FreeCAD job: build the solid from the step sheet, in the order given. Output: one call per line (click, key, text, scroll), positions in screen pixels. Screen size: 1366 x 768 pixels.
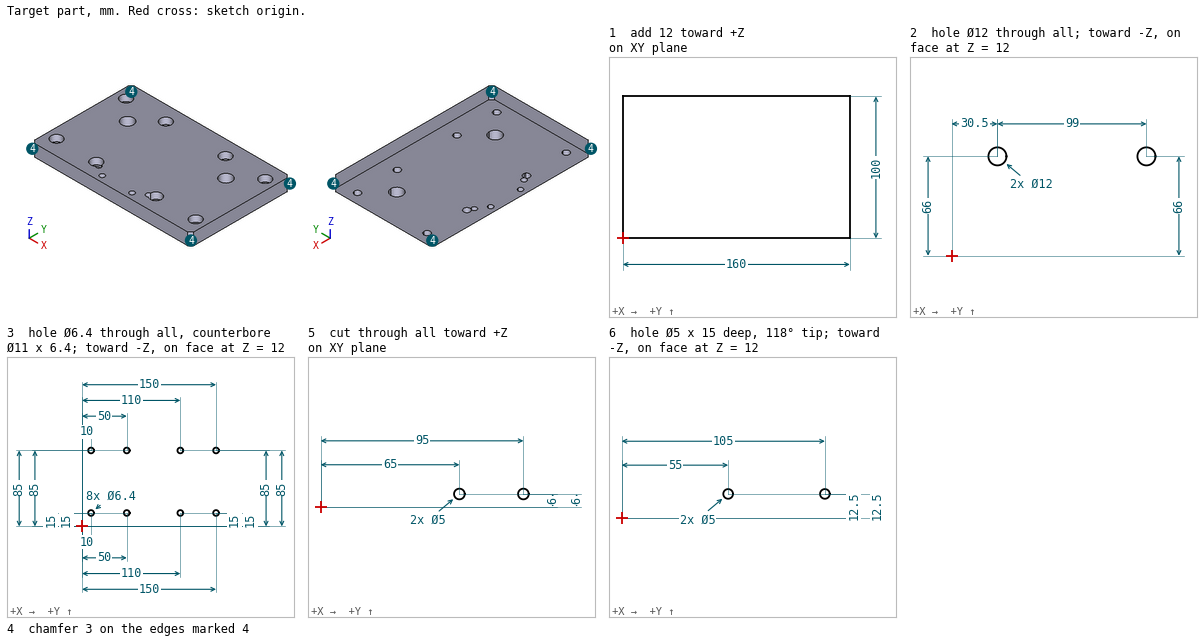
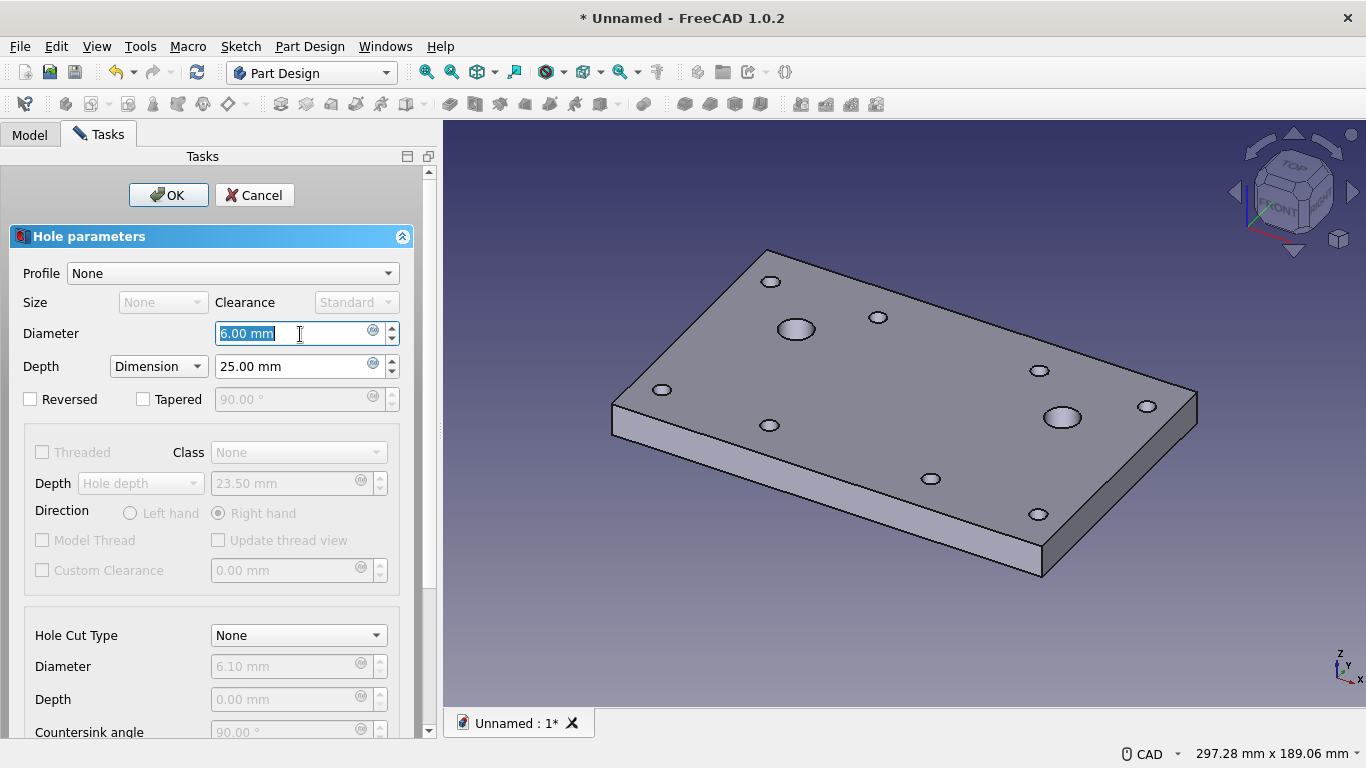
text(6.4)
key(Tab)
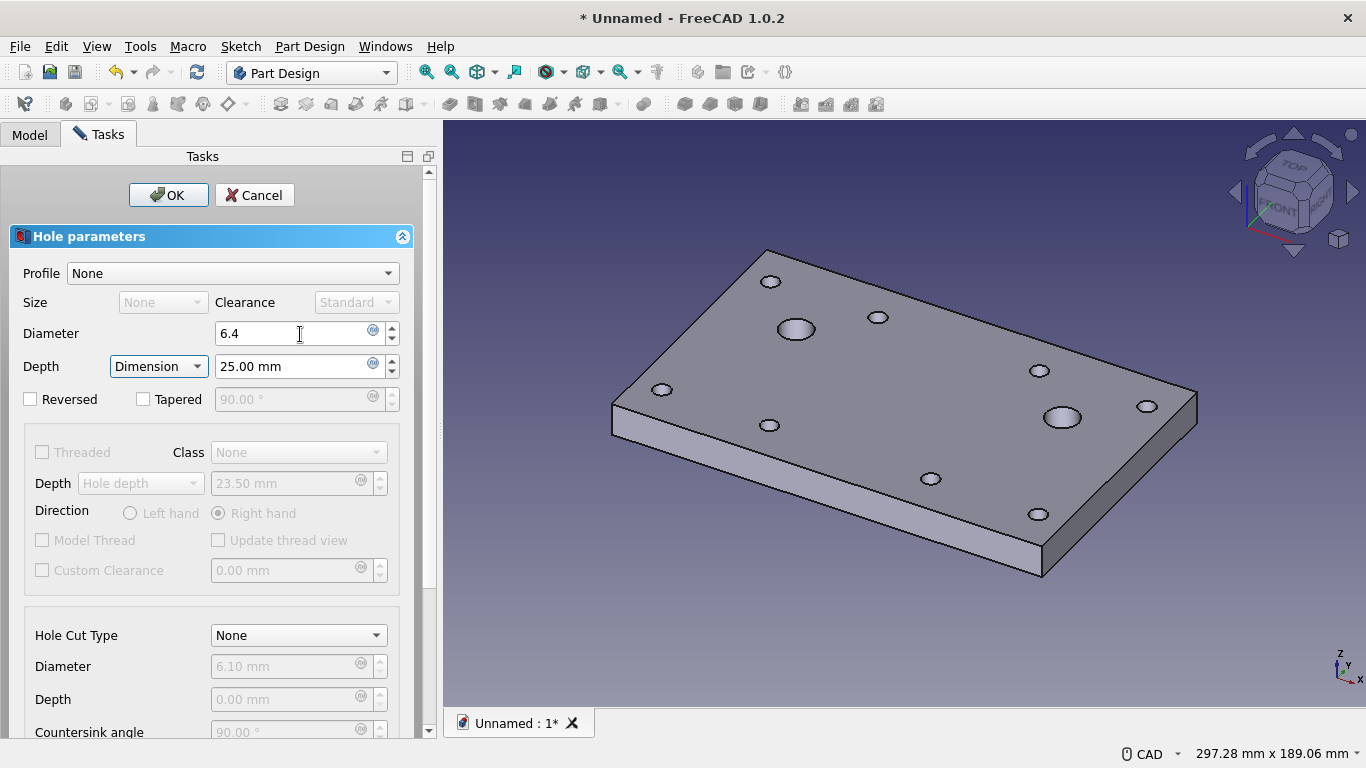
click(160, 366)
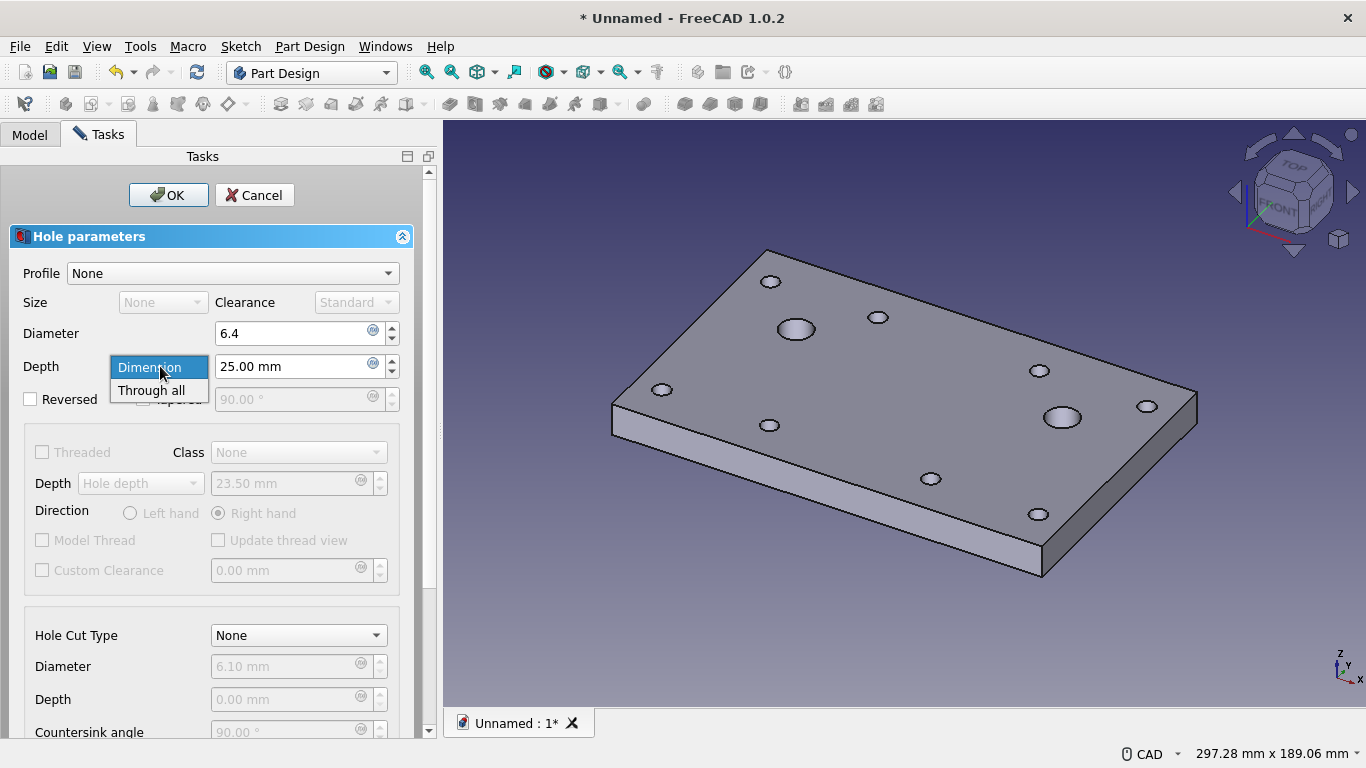
click(158, 390)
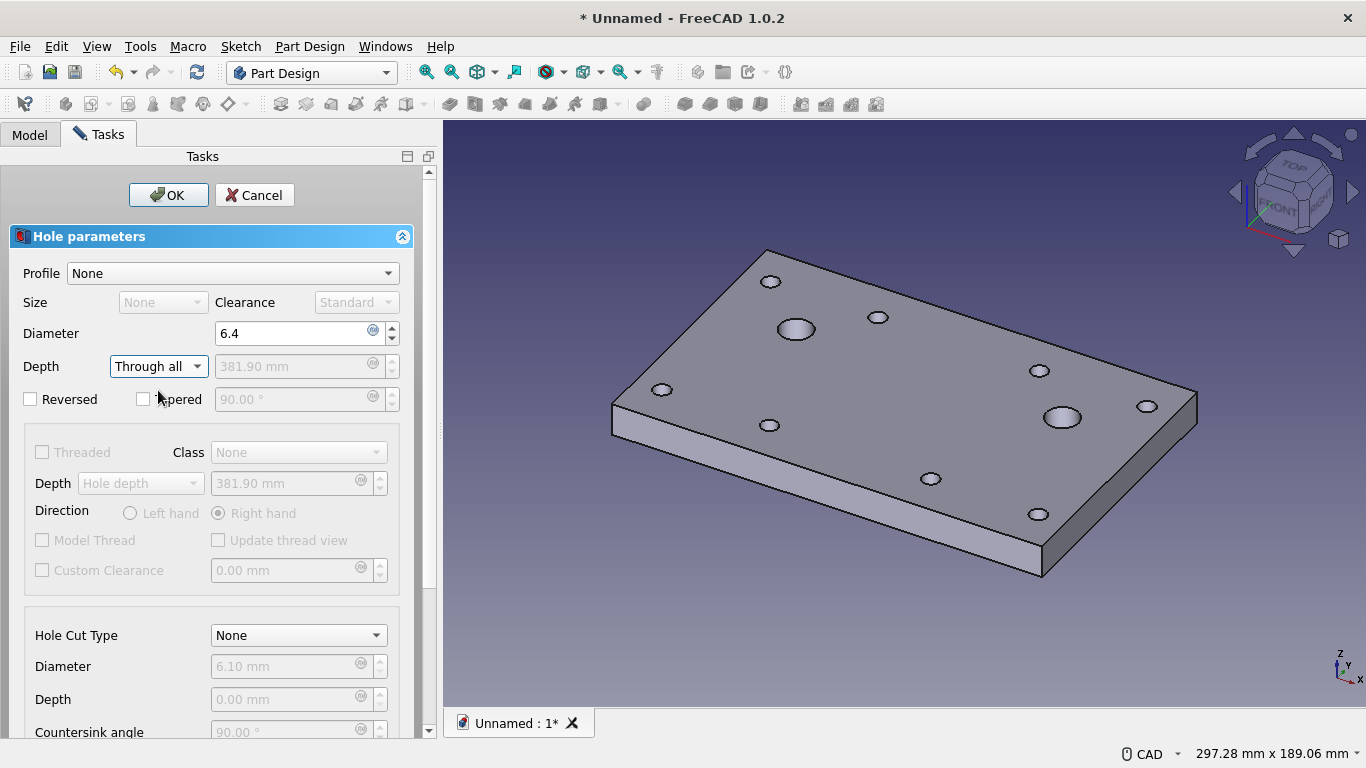
click(300, 636)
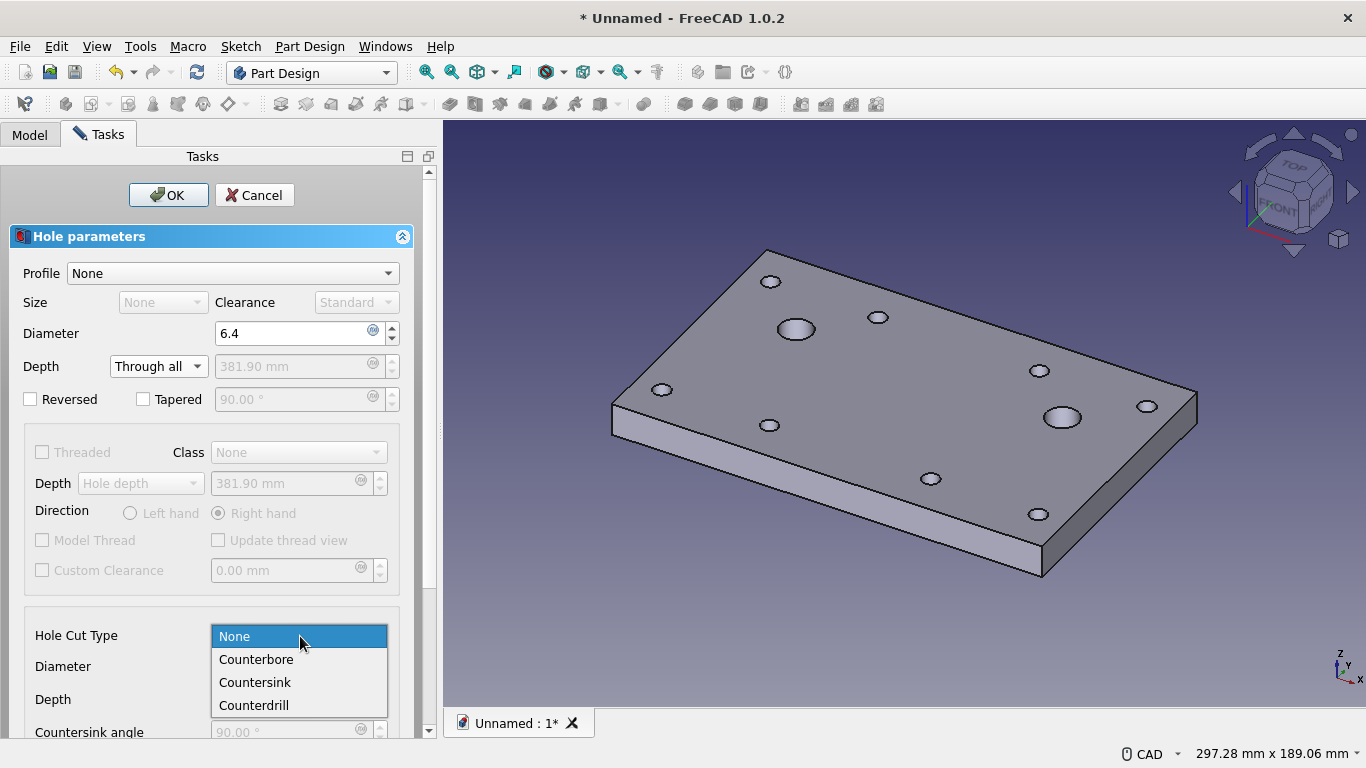
click(298, 660)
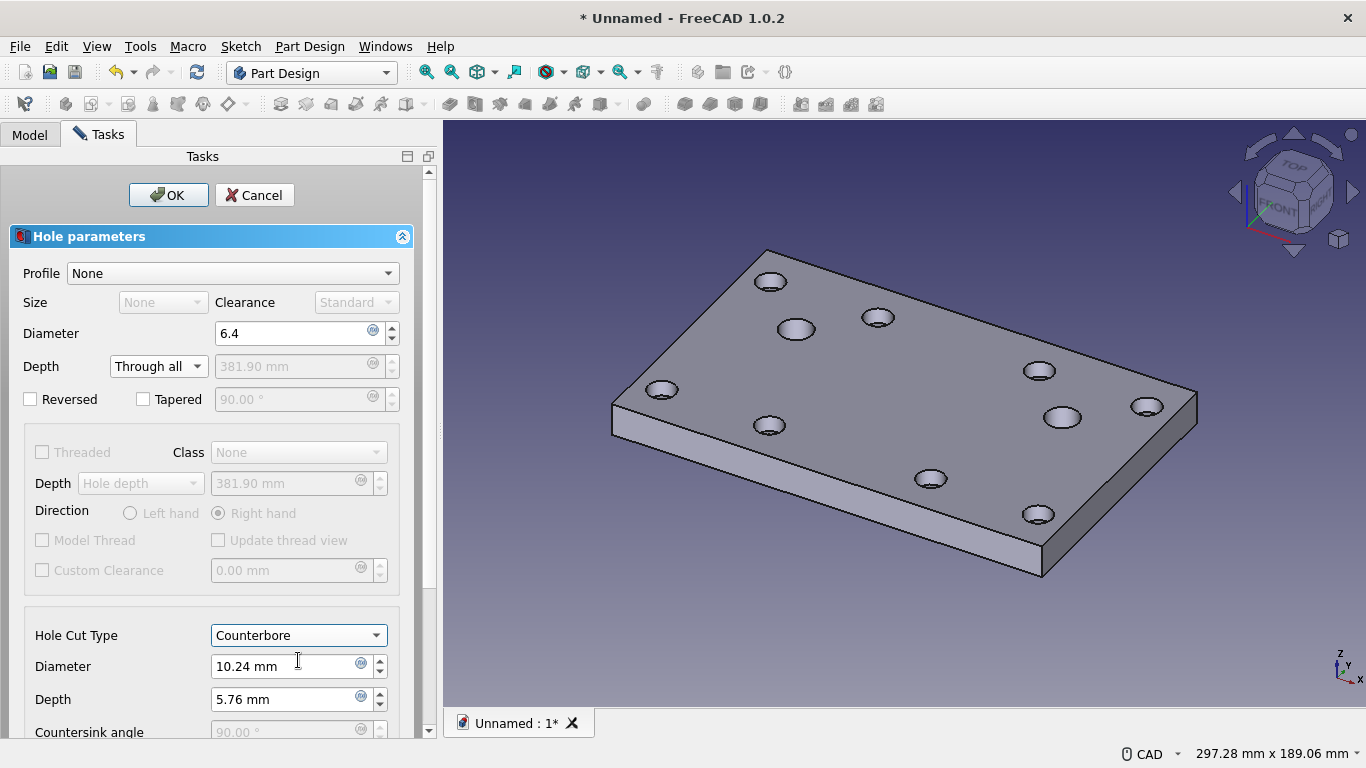
triple_click(292, 666)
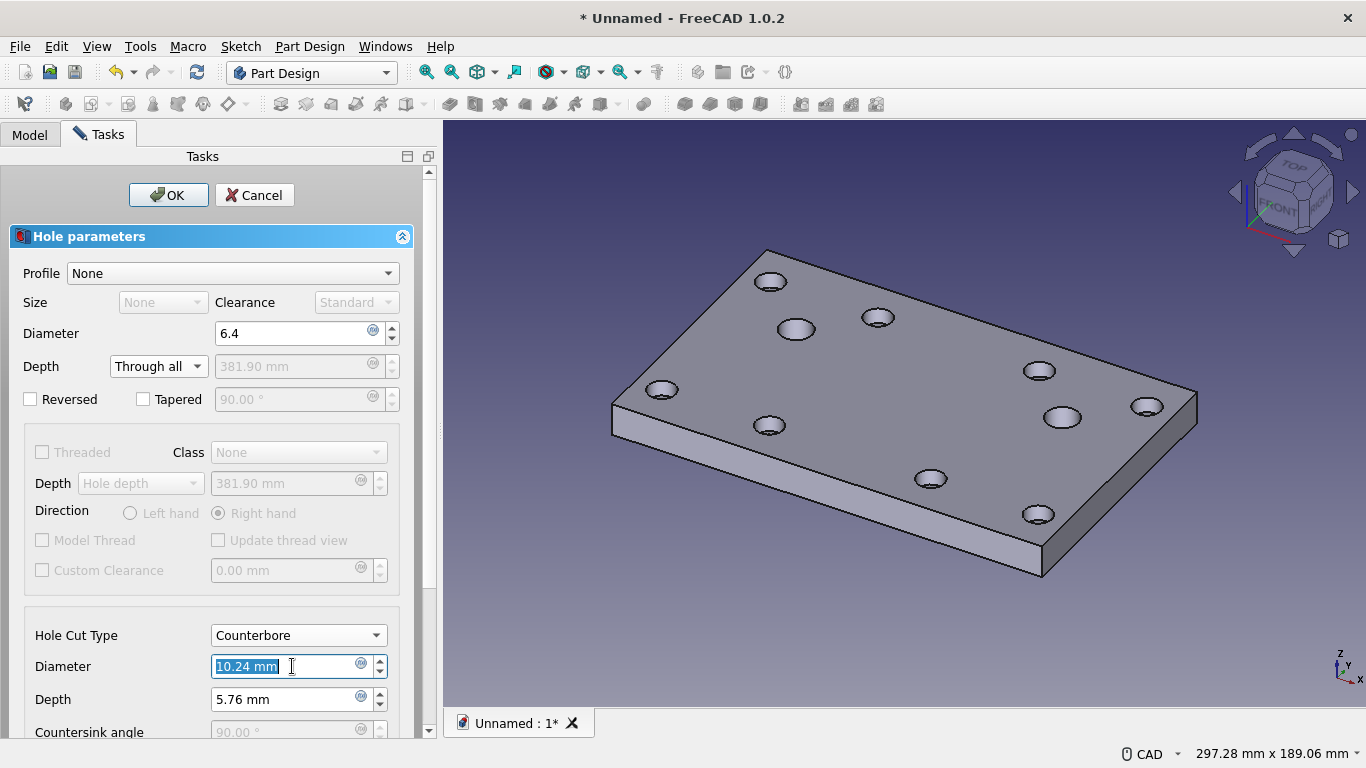
text(11)
key(Tab)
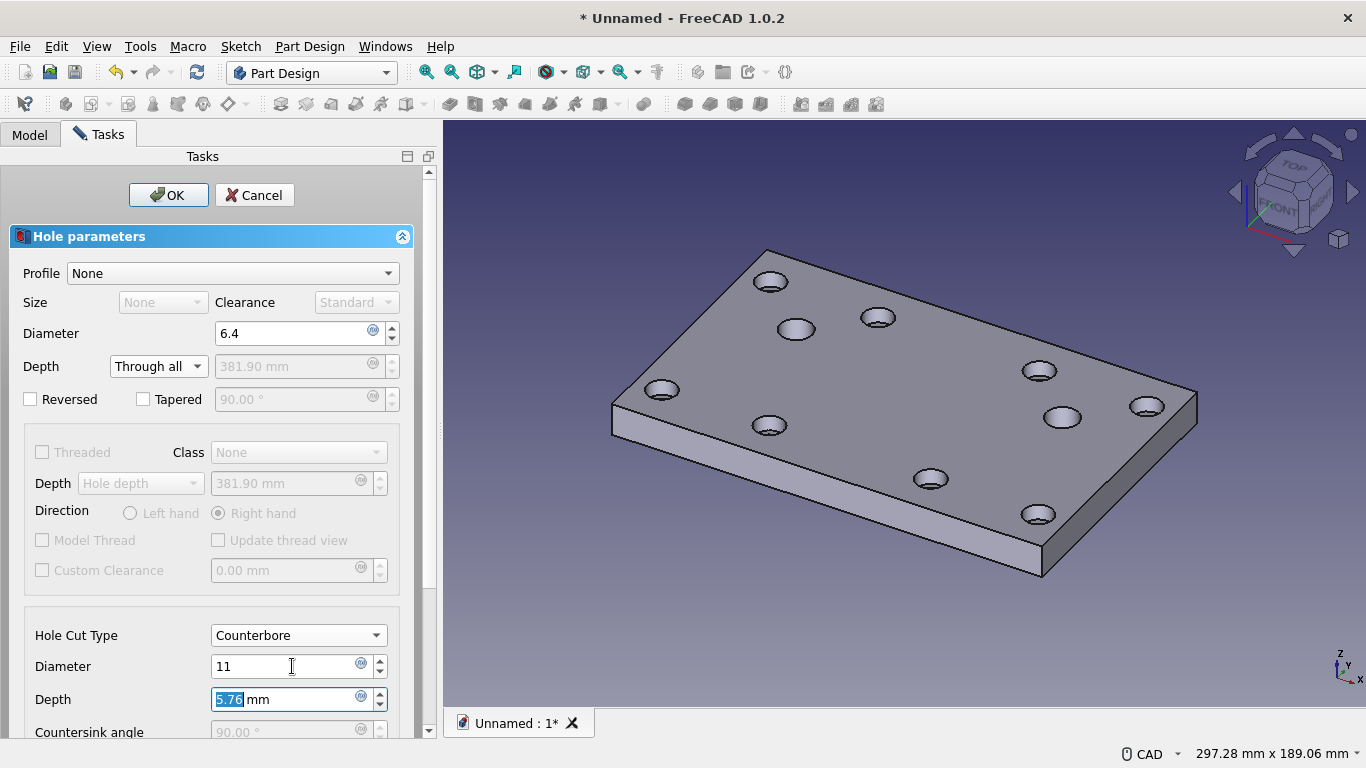
text(6.4)
key(Tab)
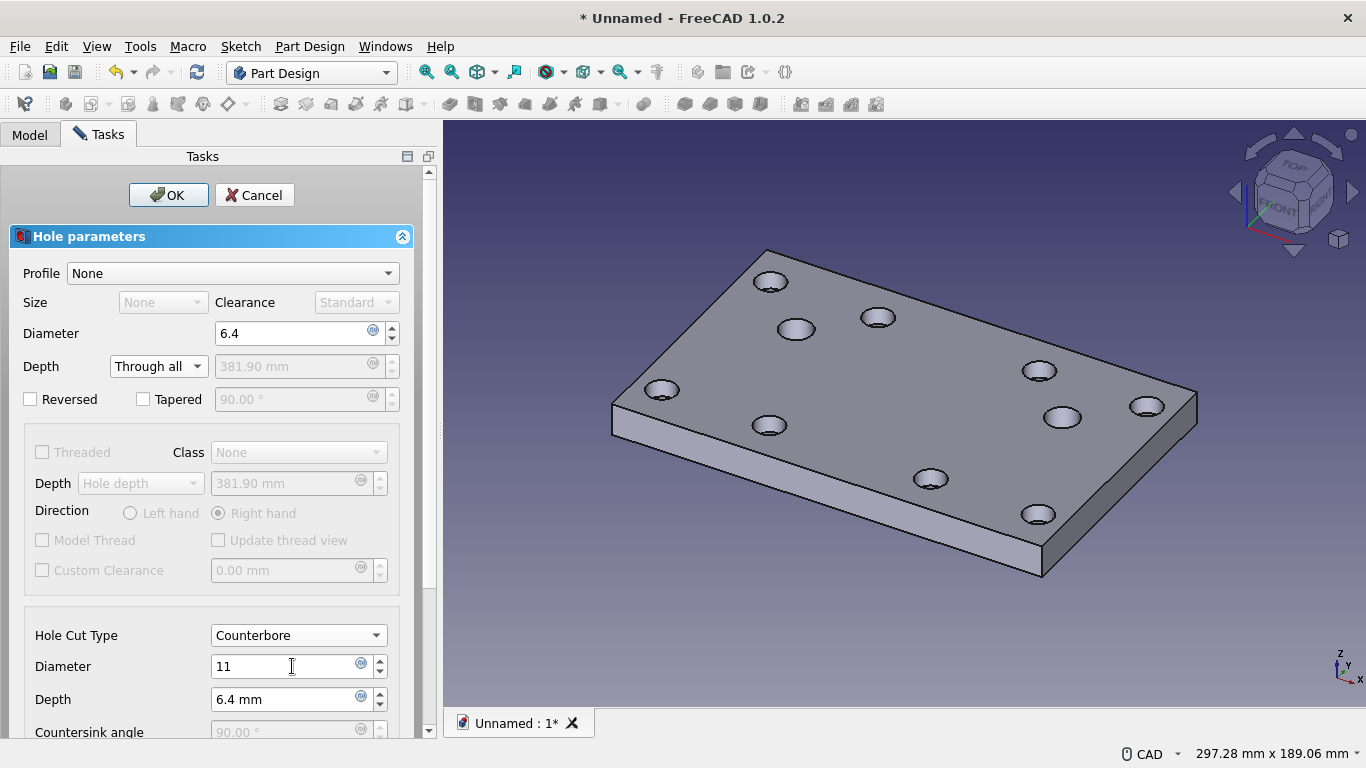
click(169, 195)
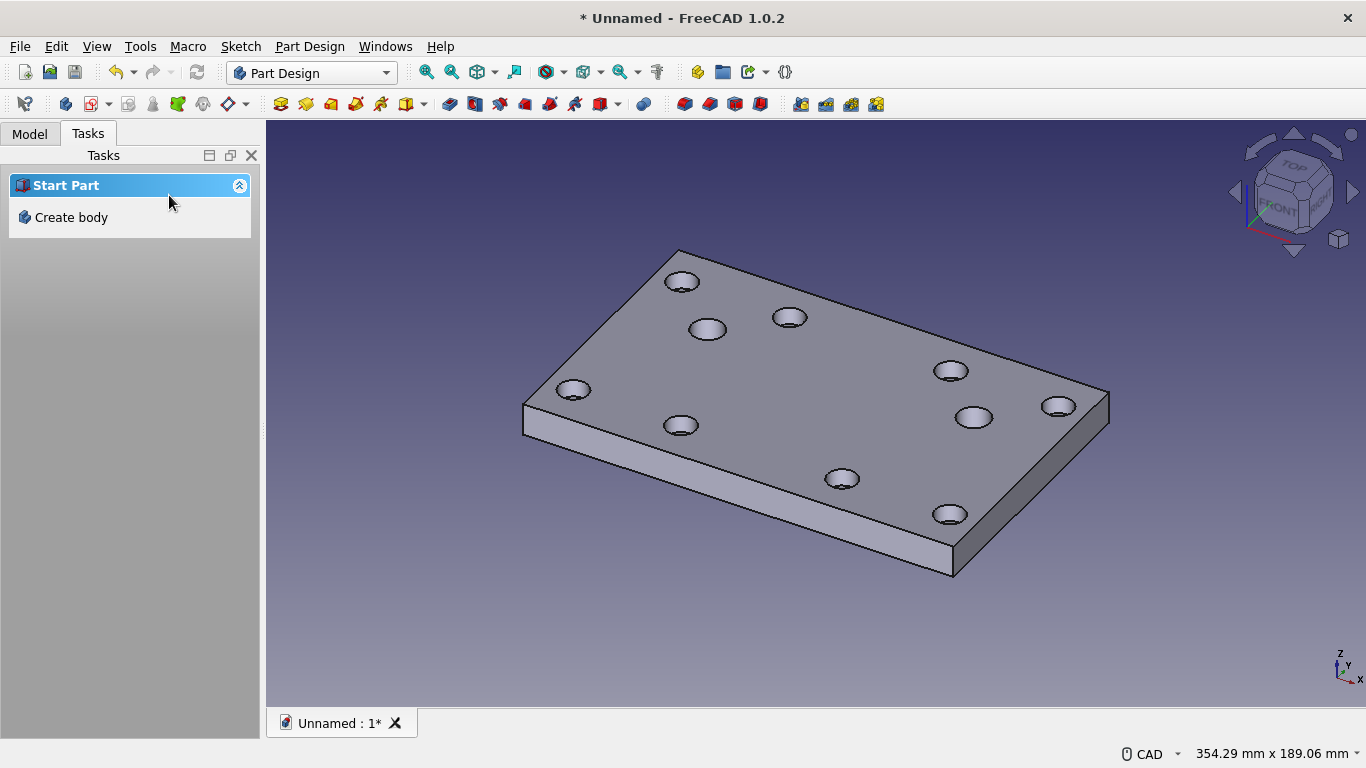
click(953, 561)